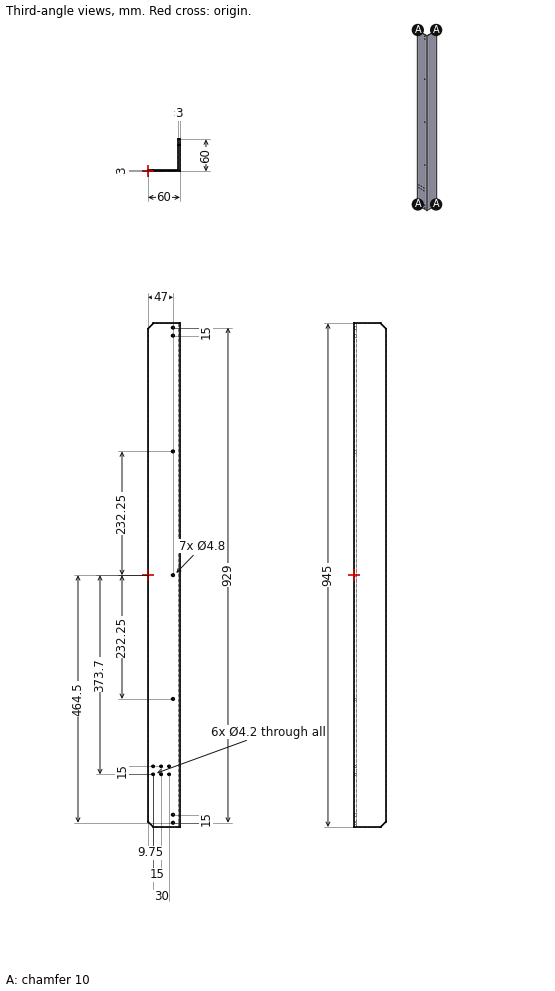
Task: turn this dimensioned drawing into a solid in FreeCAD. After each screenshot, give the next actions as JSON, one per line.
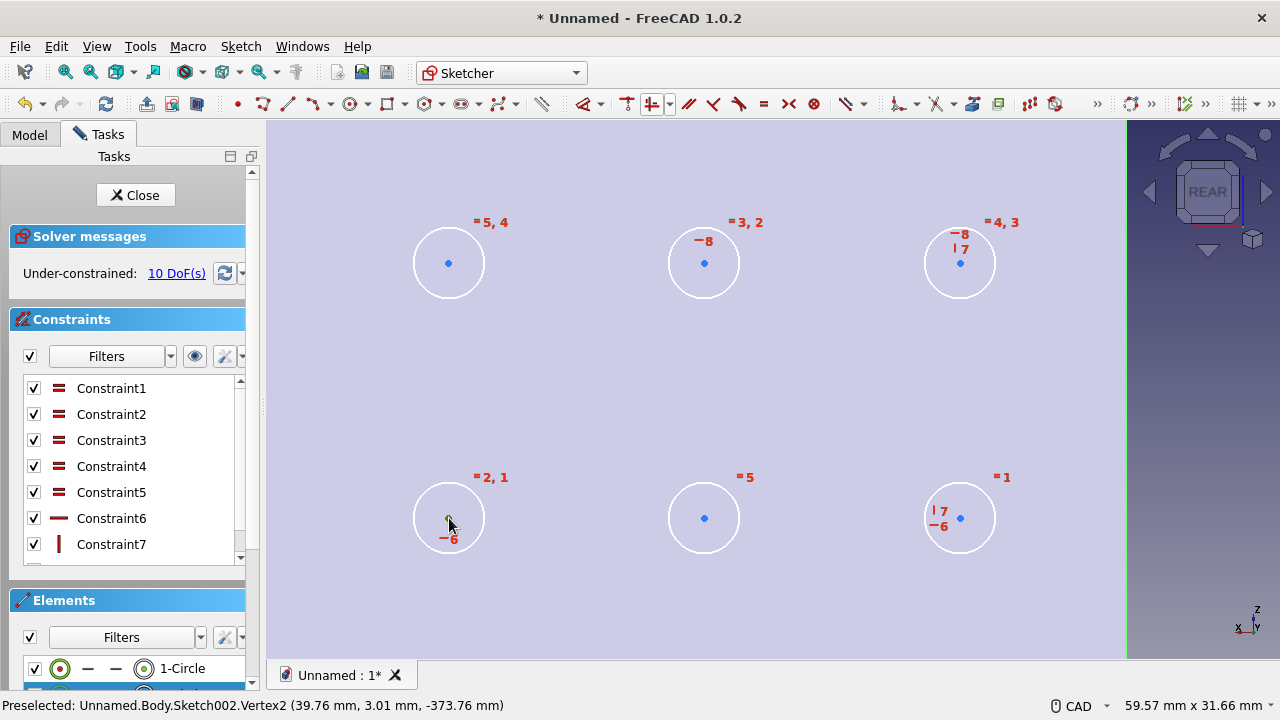
{"action": "left_click", "coordinate": [449, 263]}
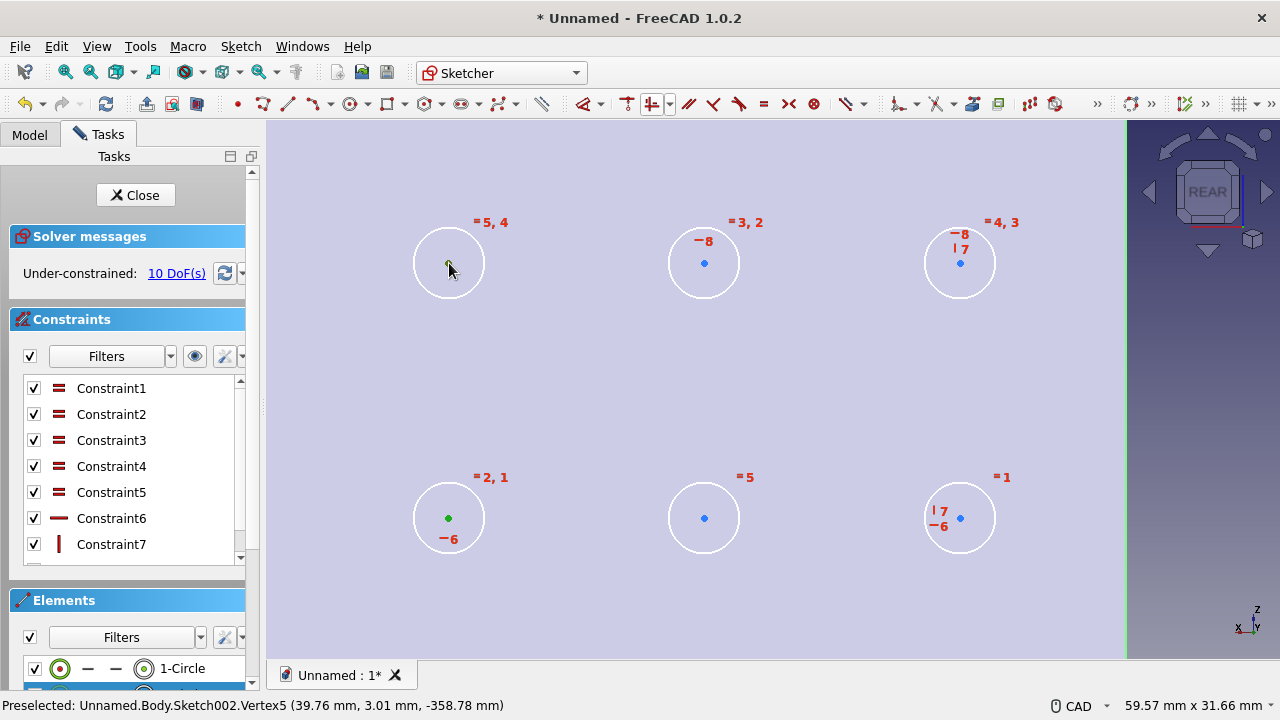
{"action": "key", "text": "v"}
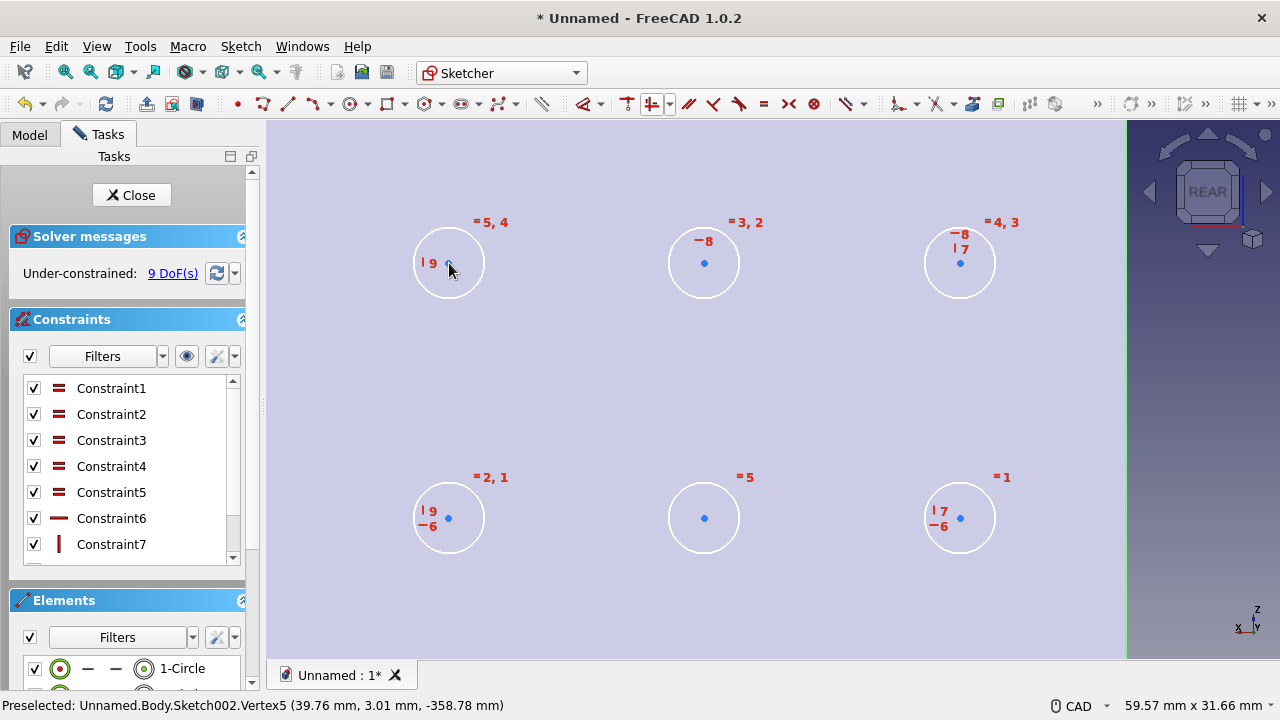
{"action": "left_click", "coordinate": [704, 263]}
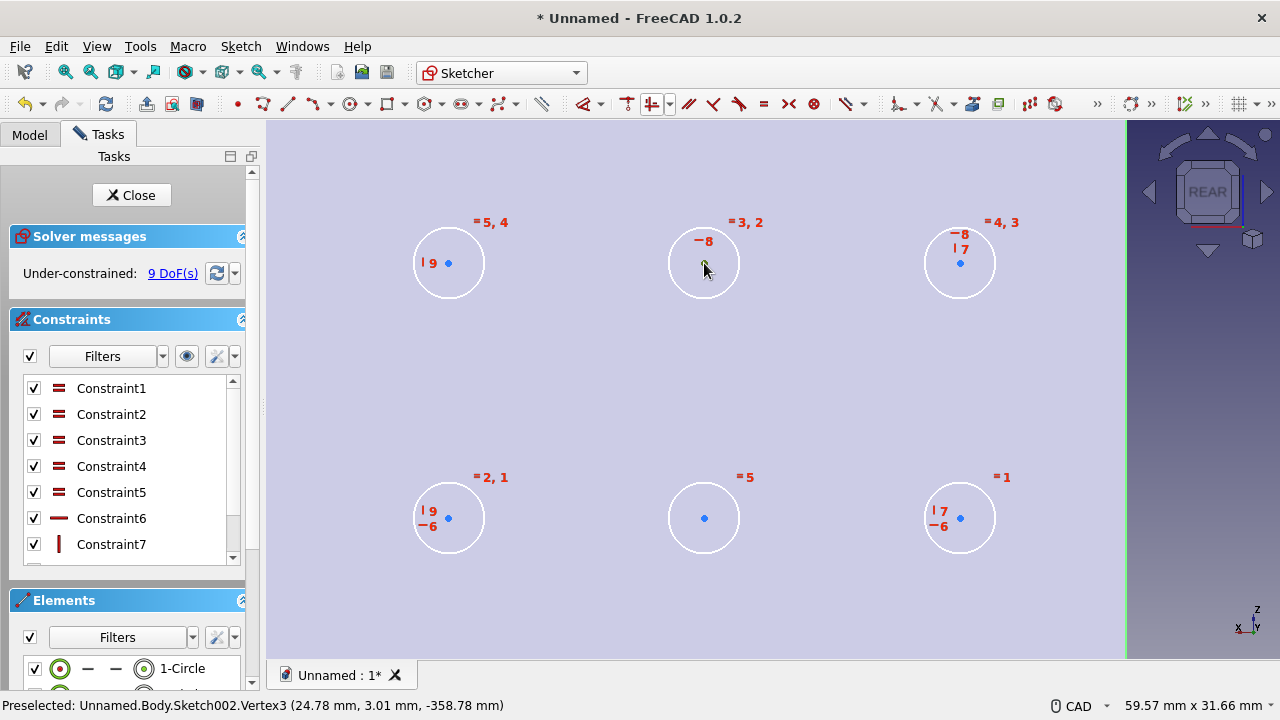
{"action": "left_click", "coordinate": [449, 263]}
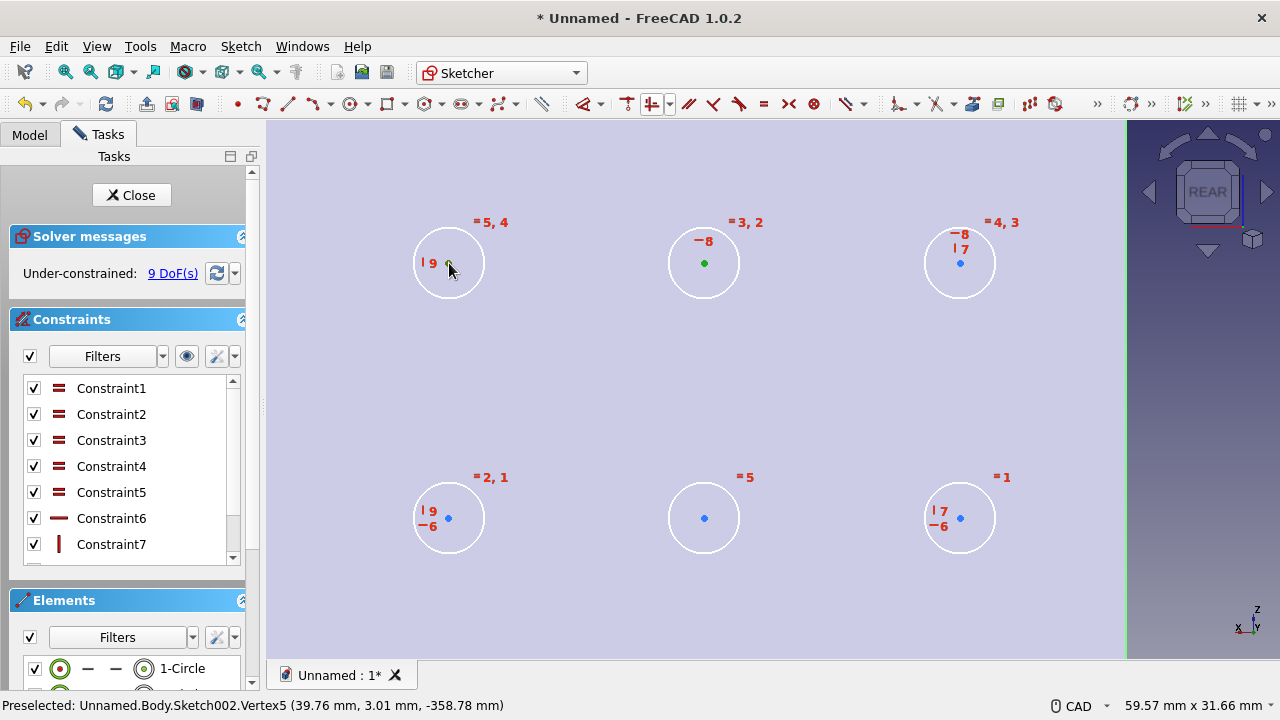
{"action": "key", "text": "h"}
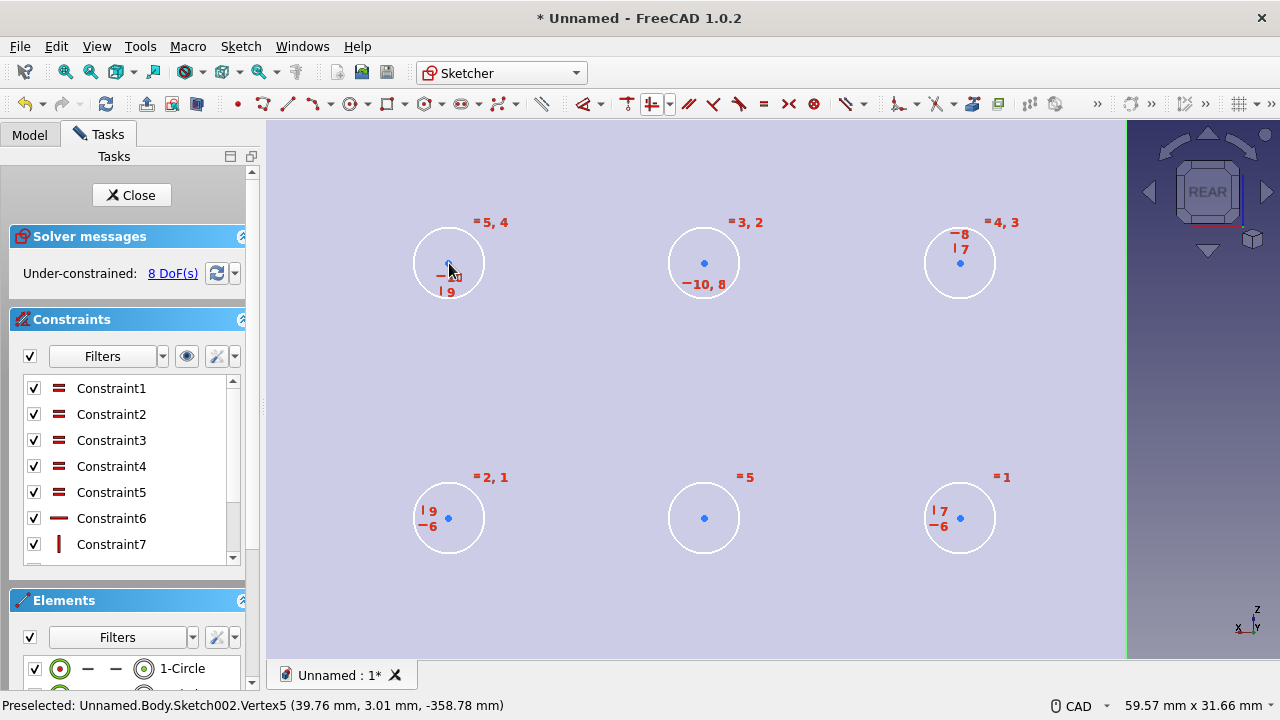
{"action": "left_click", "coordinate": [704, 263]}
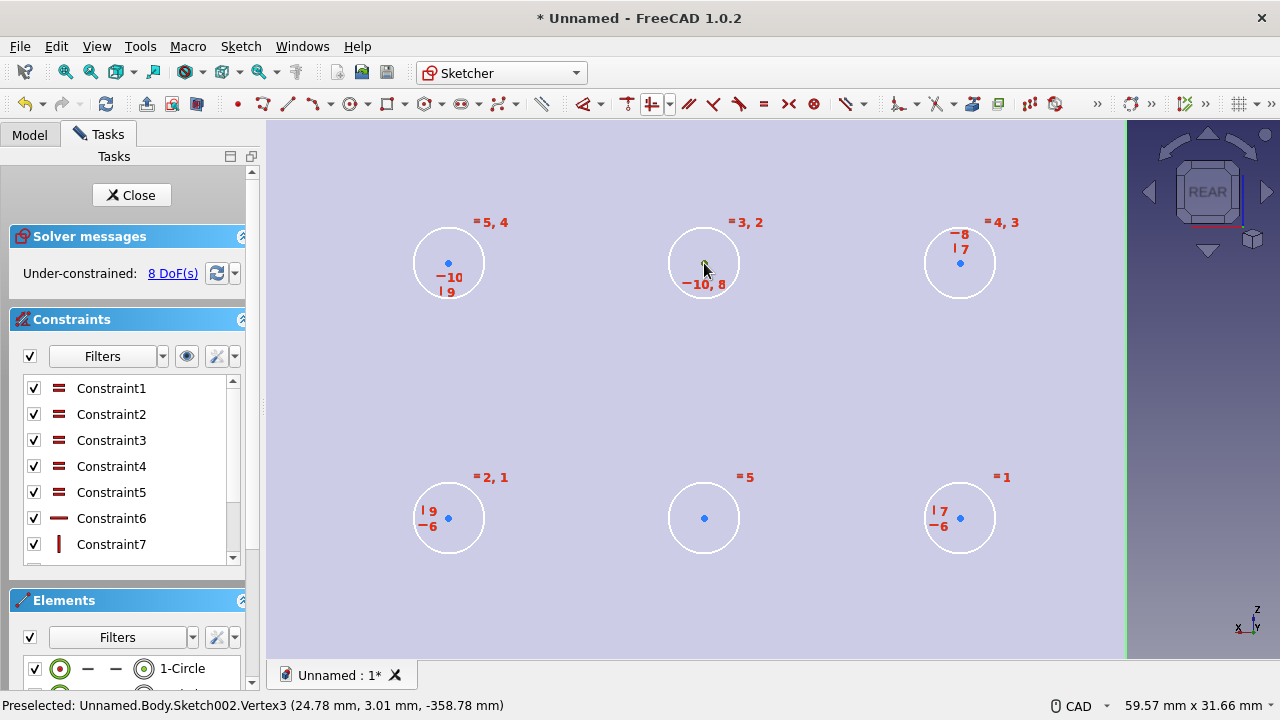
{"action": "left_click", "coordinate": [704, 518]}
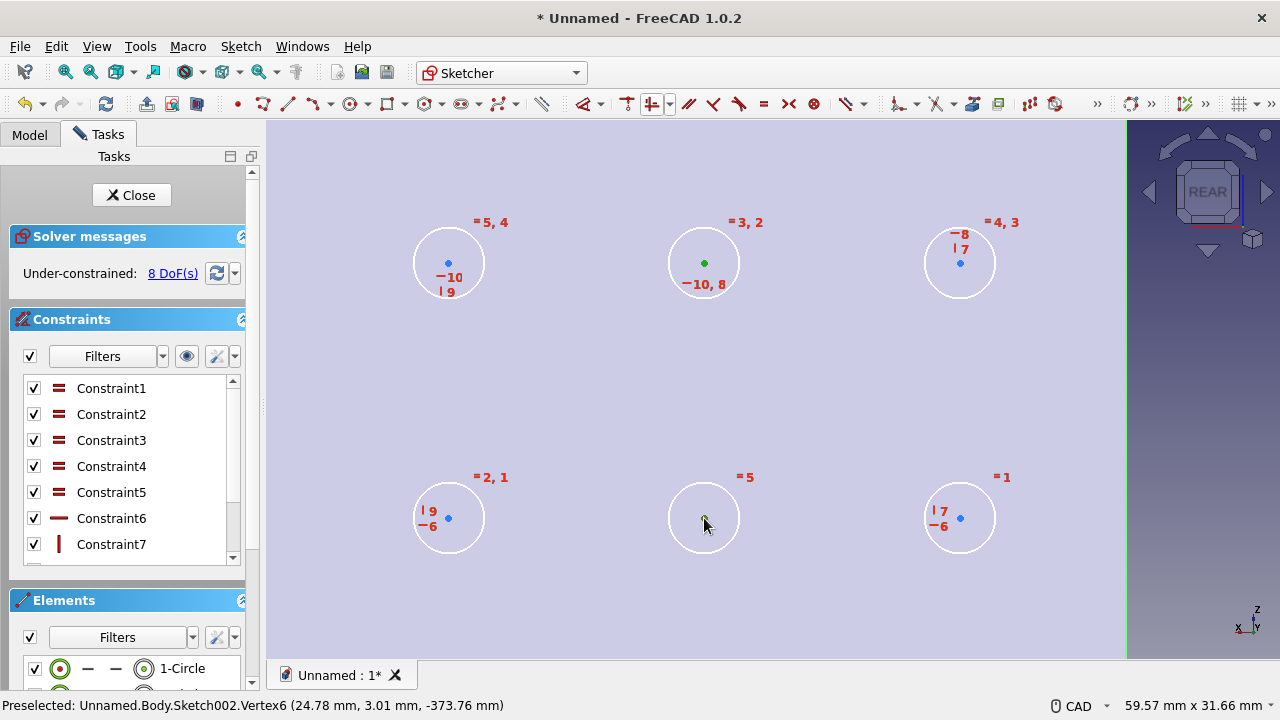
{"action": "key", "text": "v"}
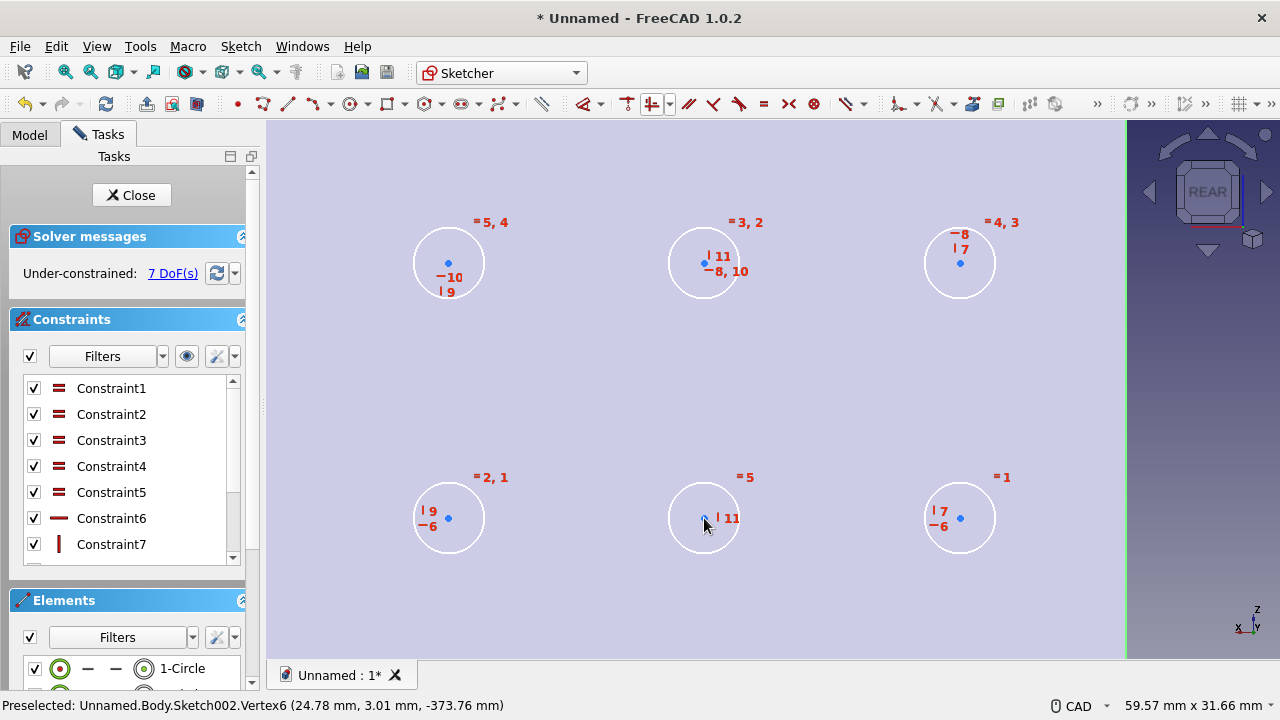
{"action": "left_click", "coordinate": [960, 518]}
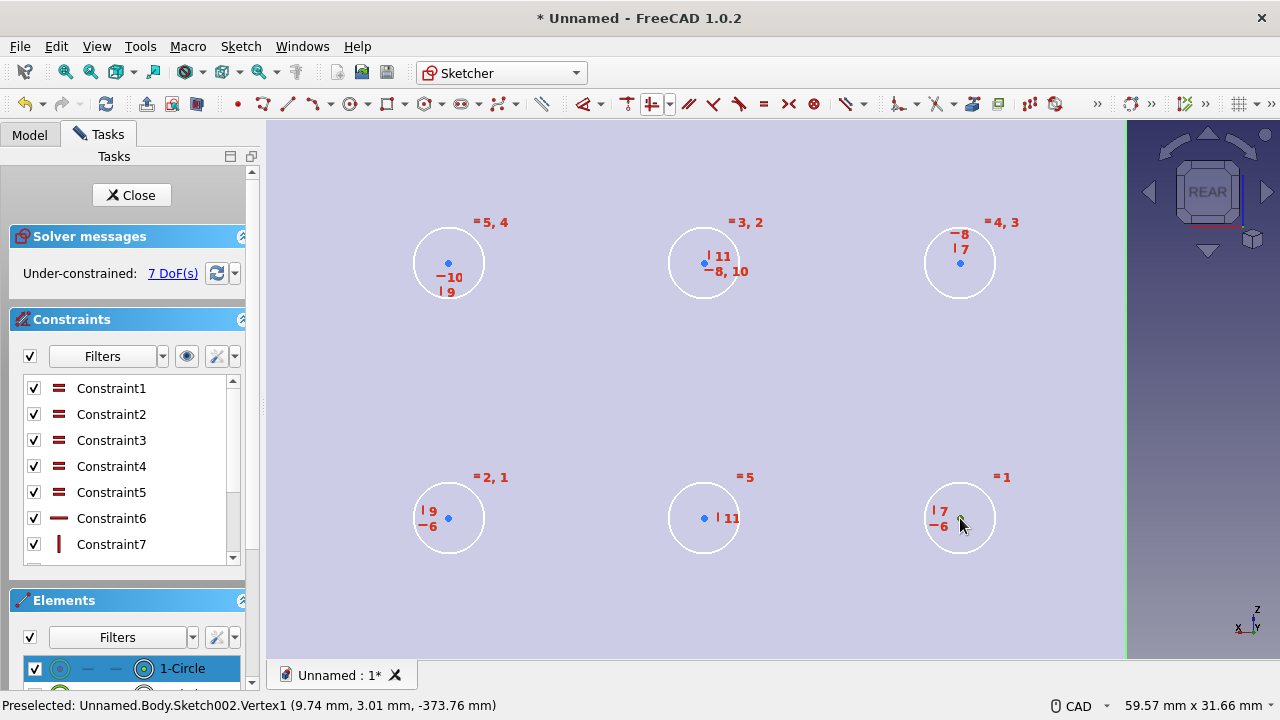
{"action": "left_click", "coordinate": [704, 518]}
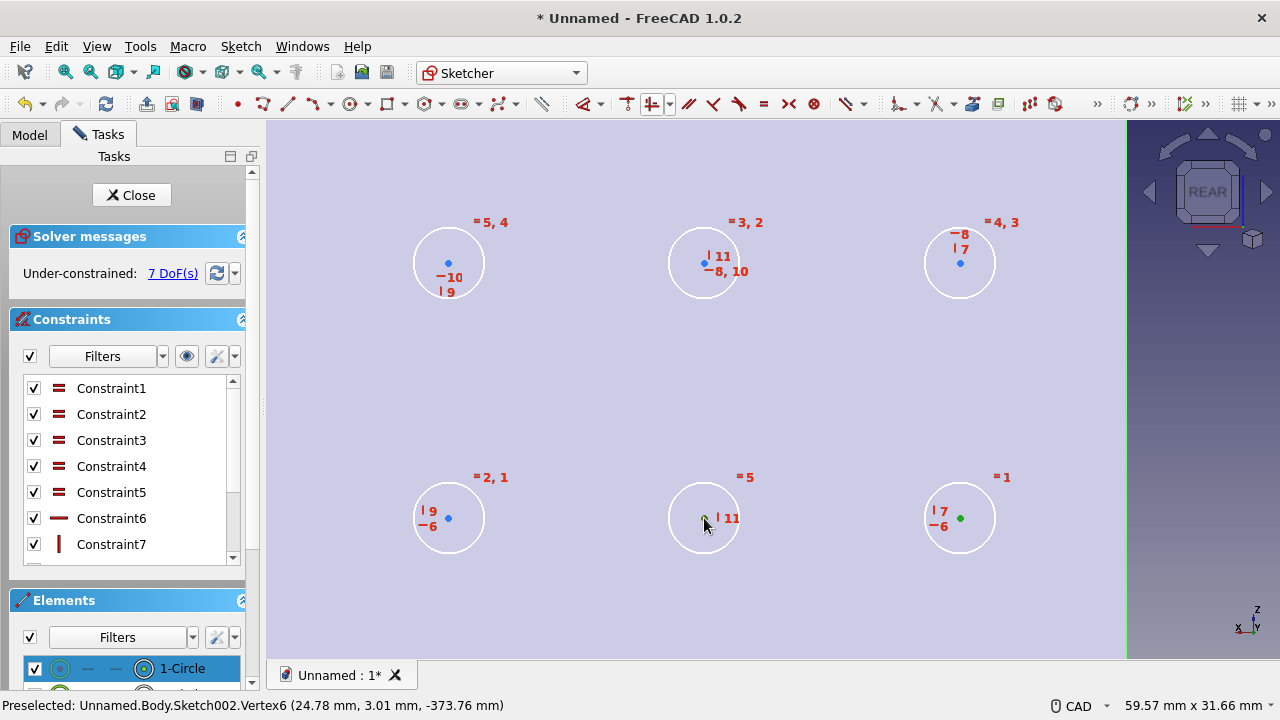
{"action": "left_click", "coordinate": [670, 104]}